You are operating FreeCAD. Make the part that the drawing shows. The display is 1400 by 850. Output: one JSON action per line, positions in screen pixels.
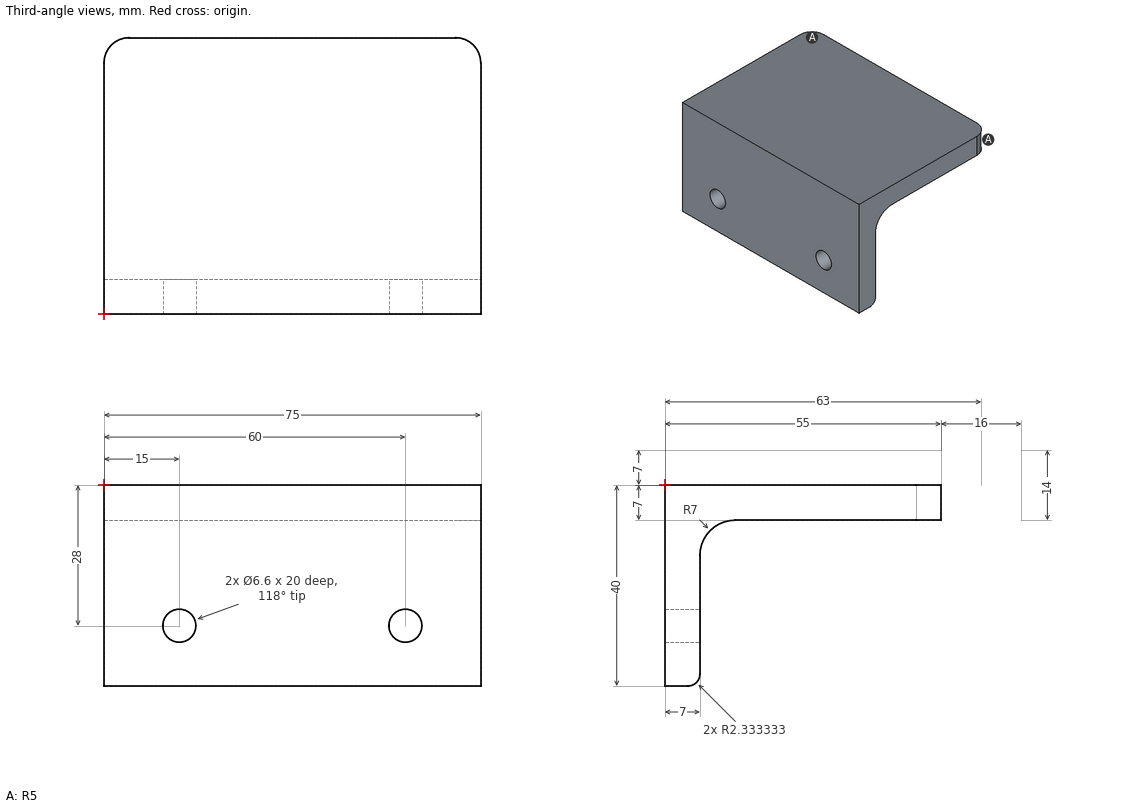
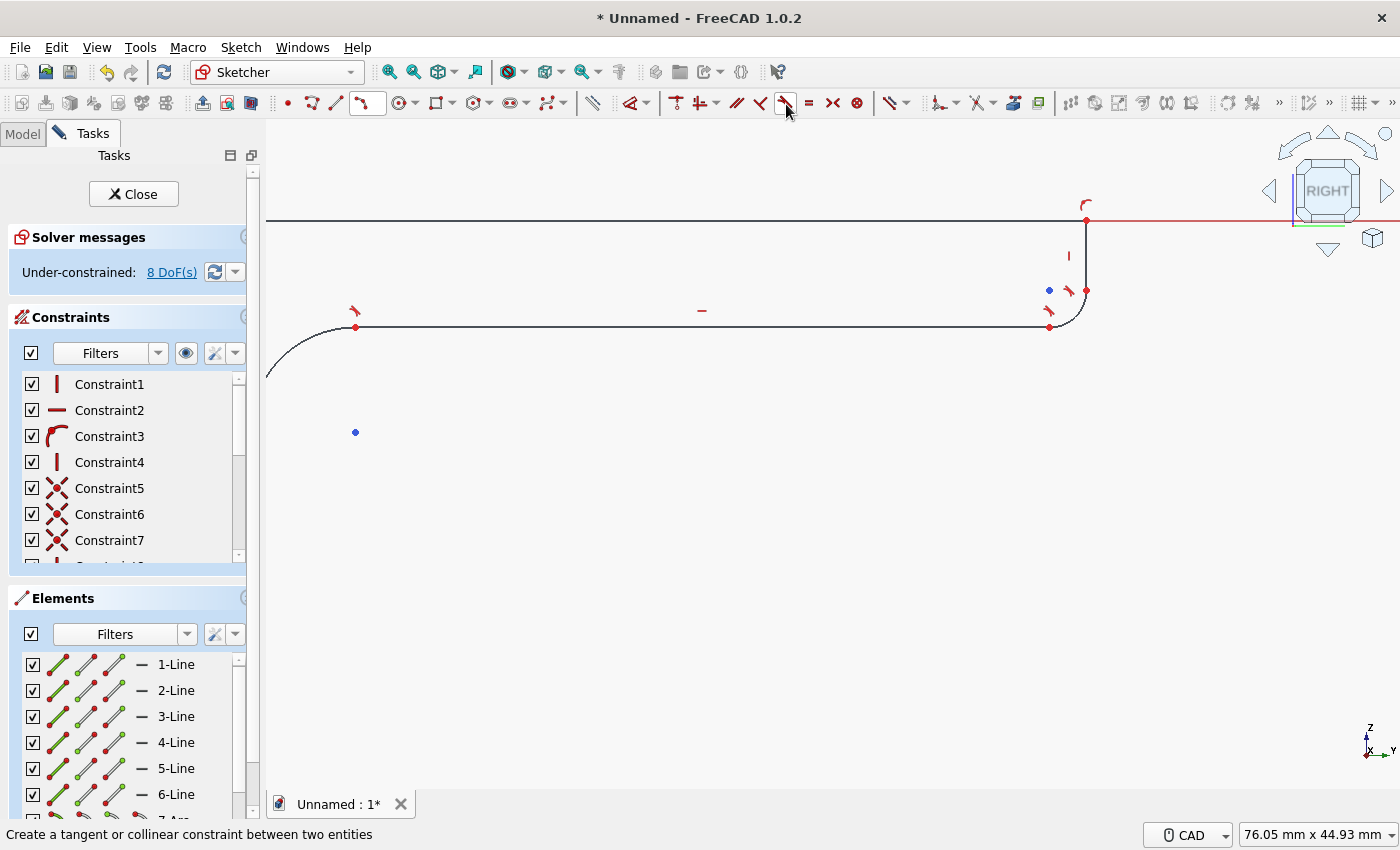
{"action": "scroll", "coordinate": [1066, 322], "scroll_direction": "down", "scroll_amount": 2}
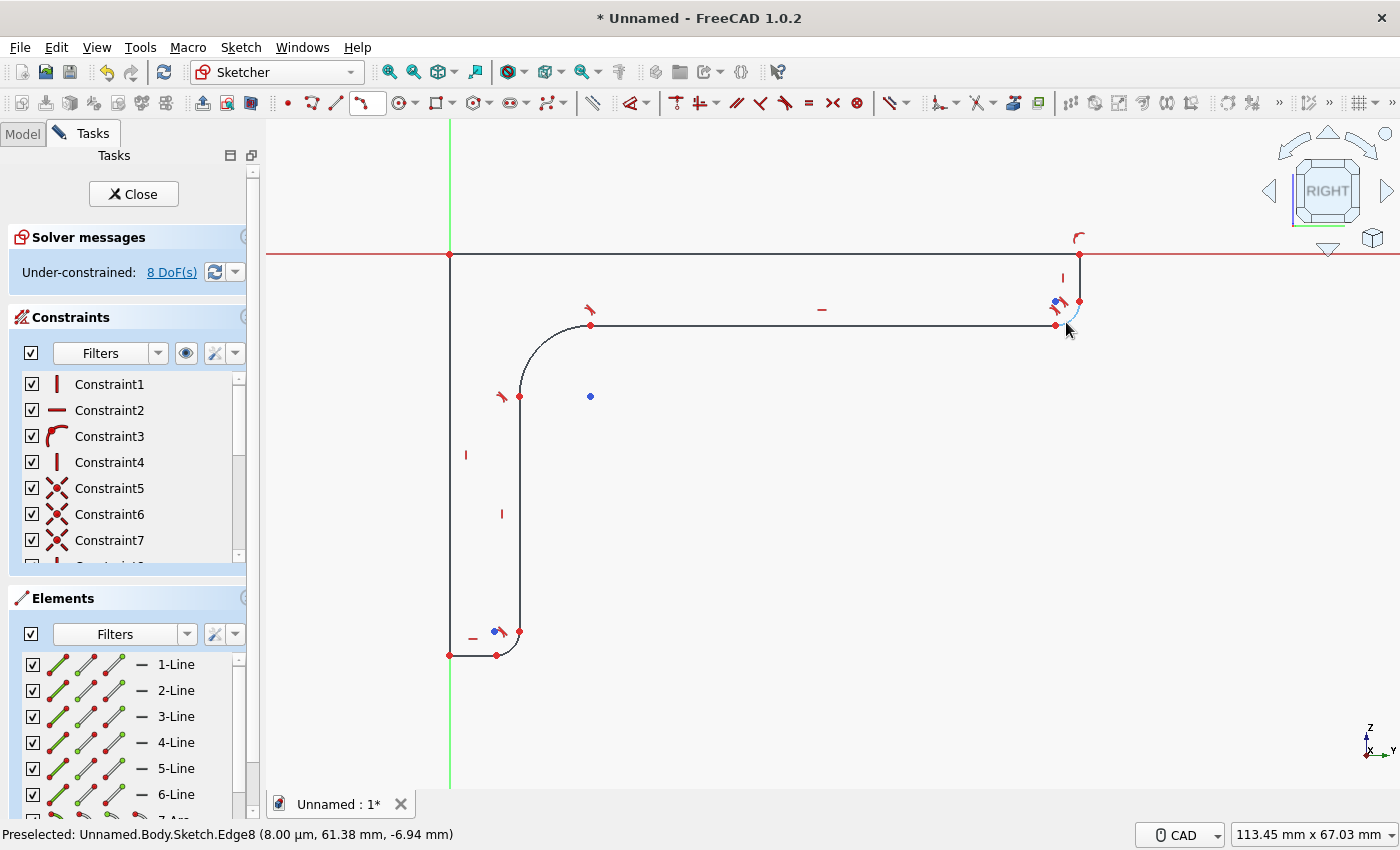
{"action": "left_click", "coordinate": [464, 656]}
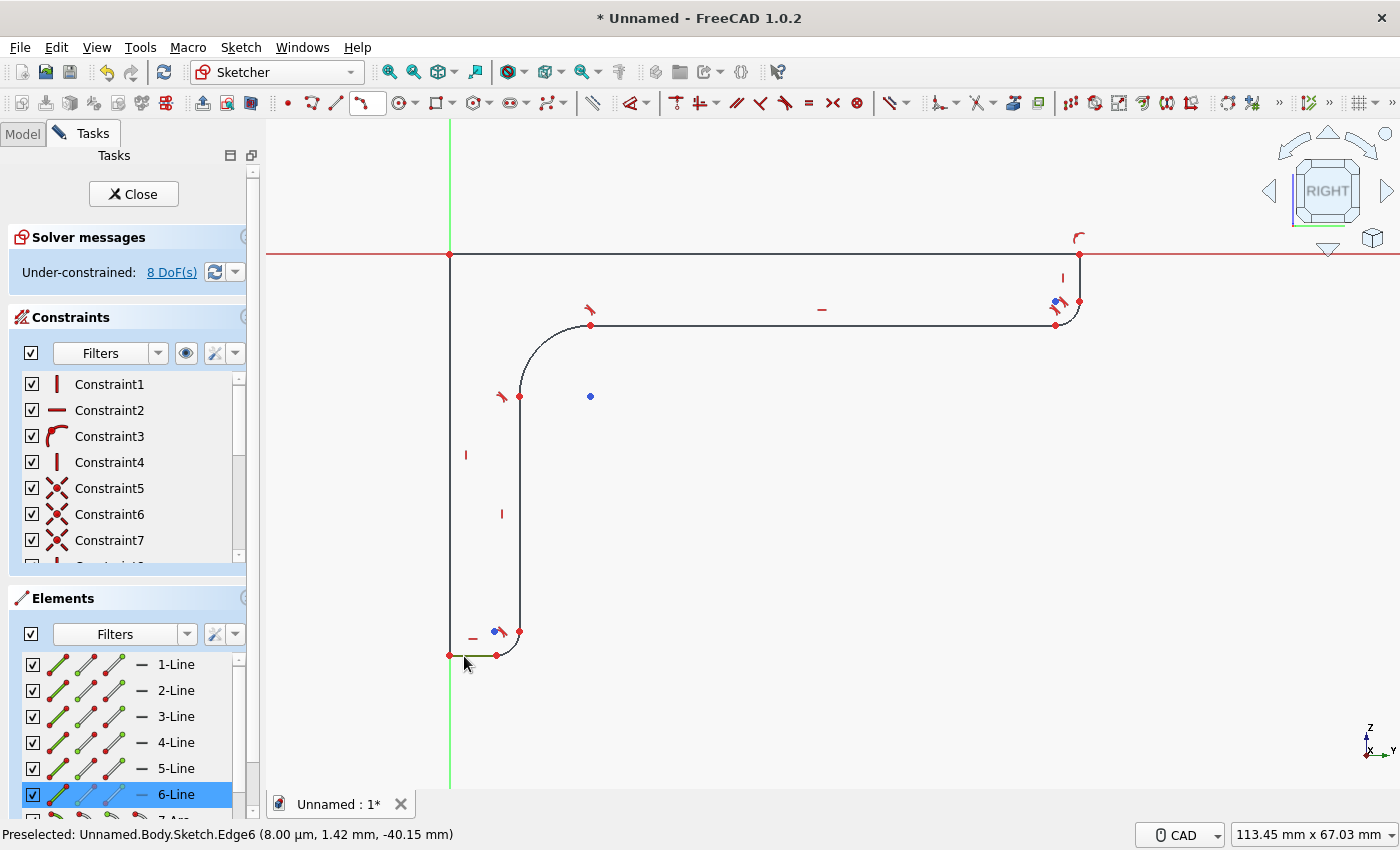
{"action": "scroll", "coordinate": [507, 652], "scroll_direction": "up", "scroll_amount": 2}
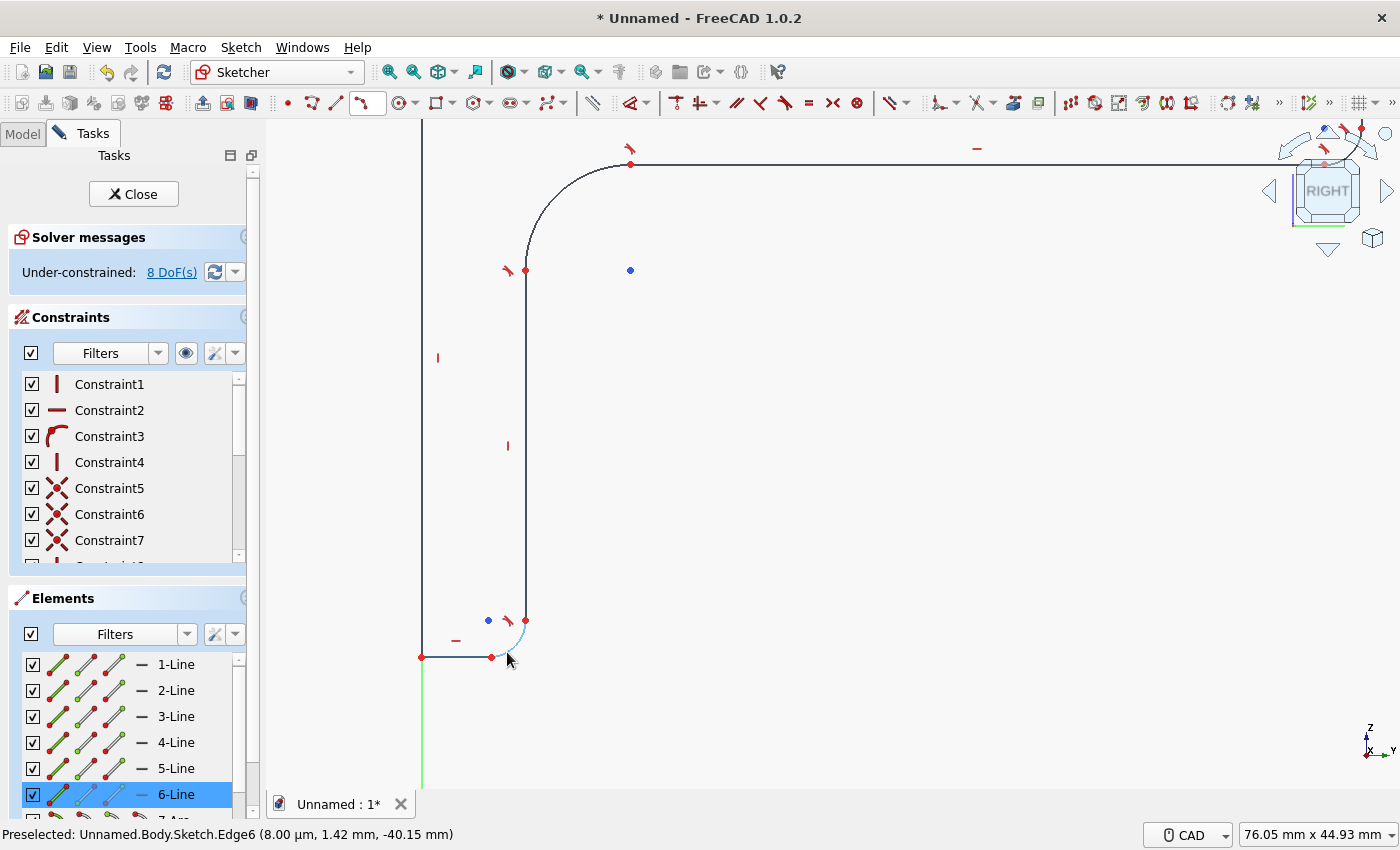
{"action": "left_click", "coordinate": [507, 652]}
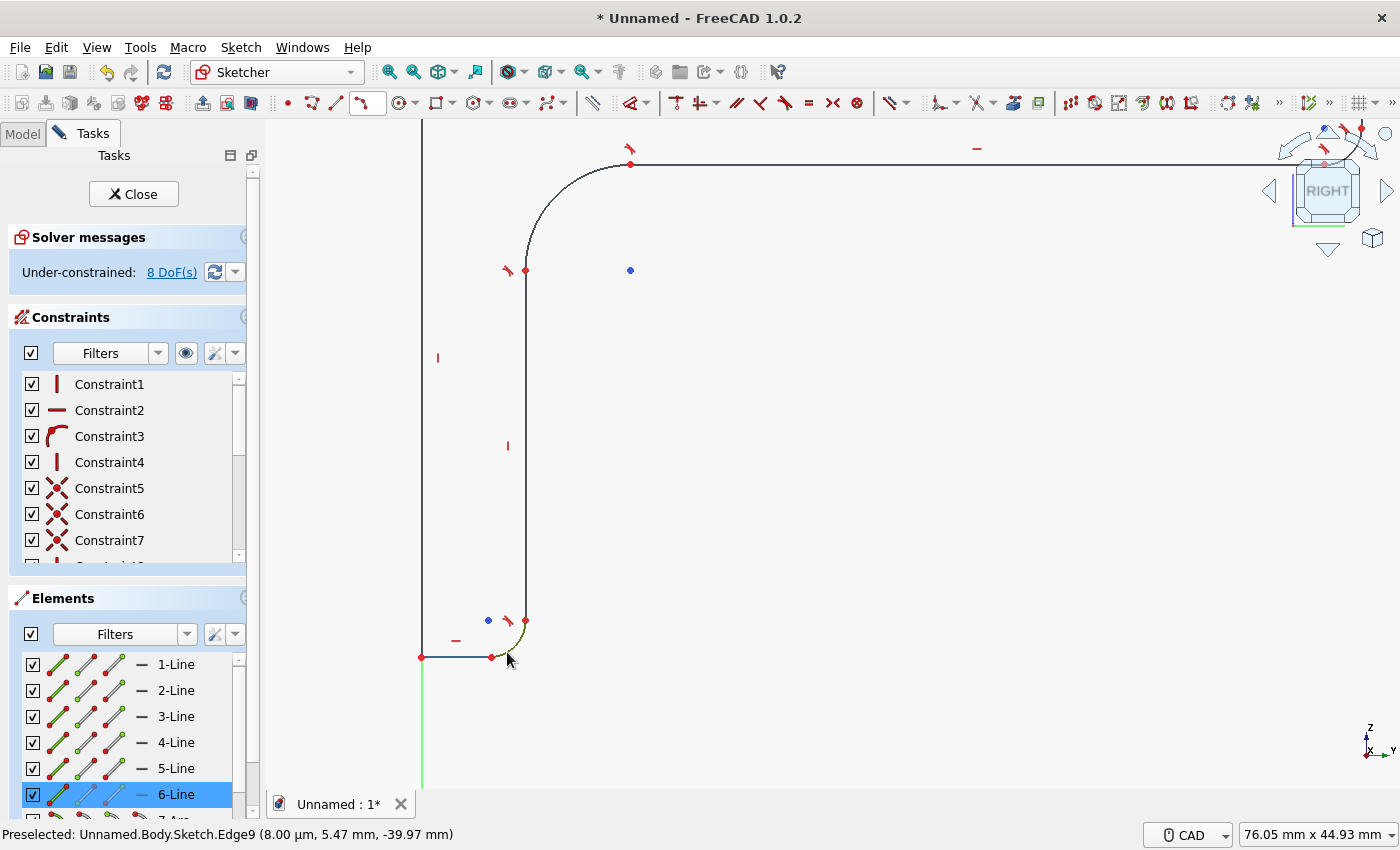
{"action": "key", "text": "t"}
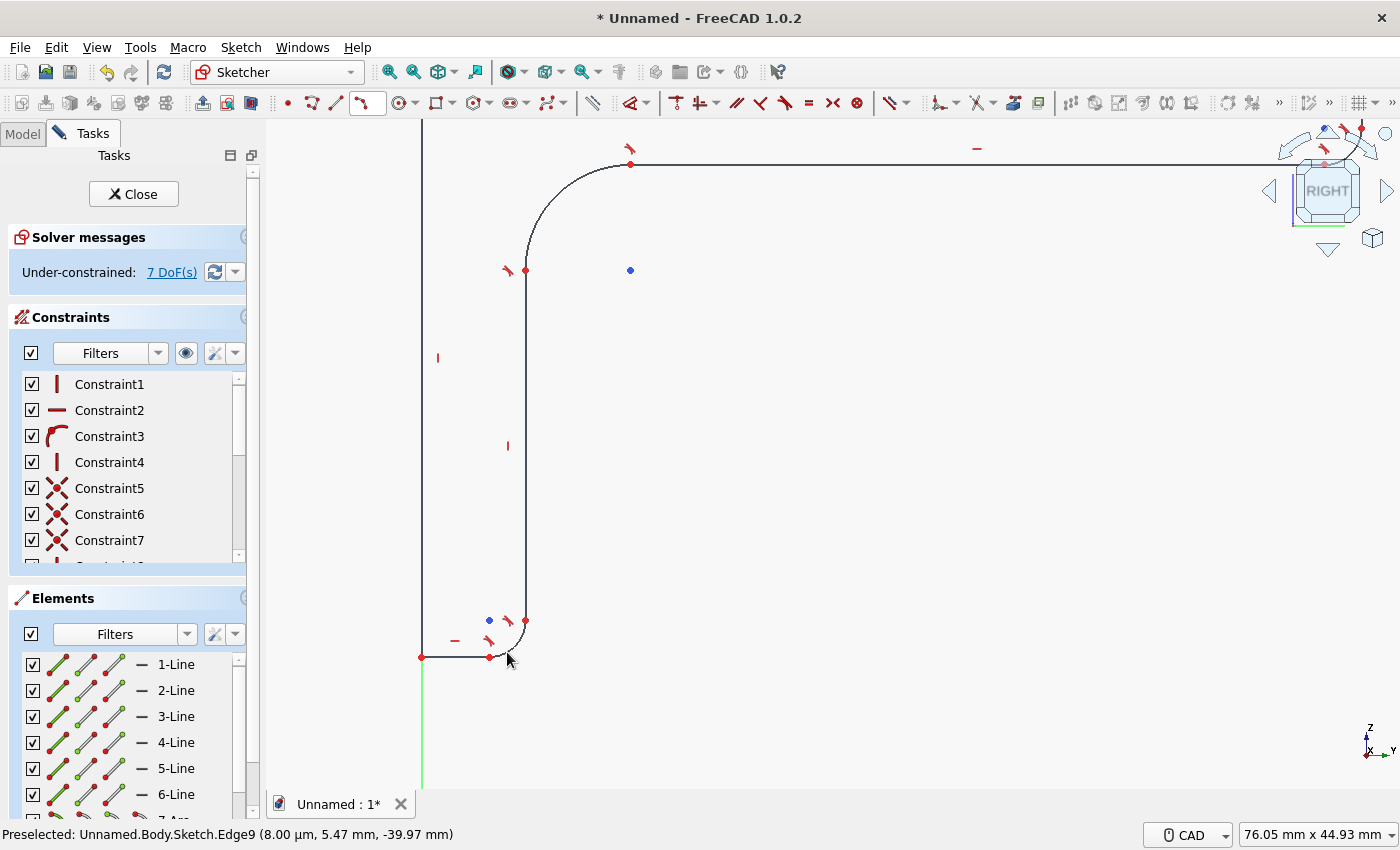
{"action": "scroll", "coordinate": [507, 652], "scroll_direction": "down", "scroll_amount": 2}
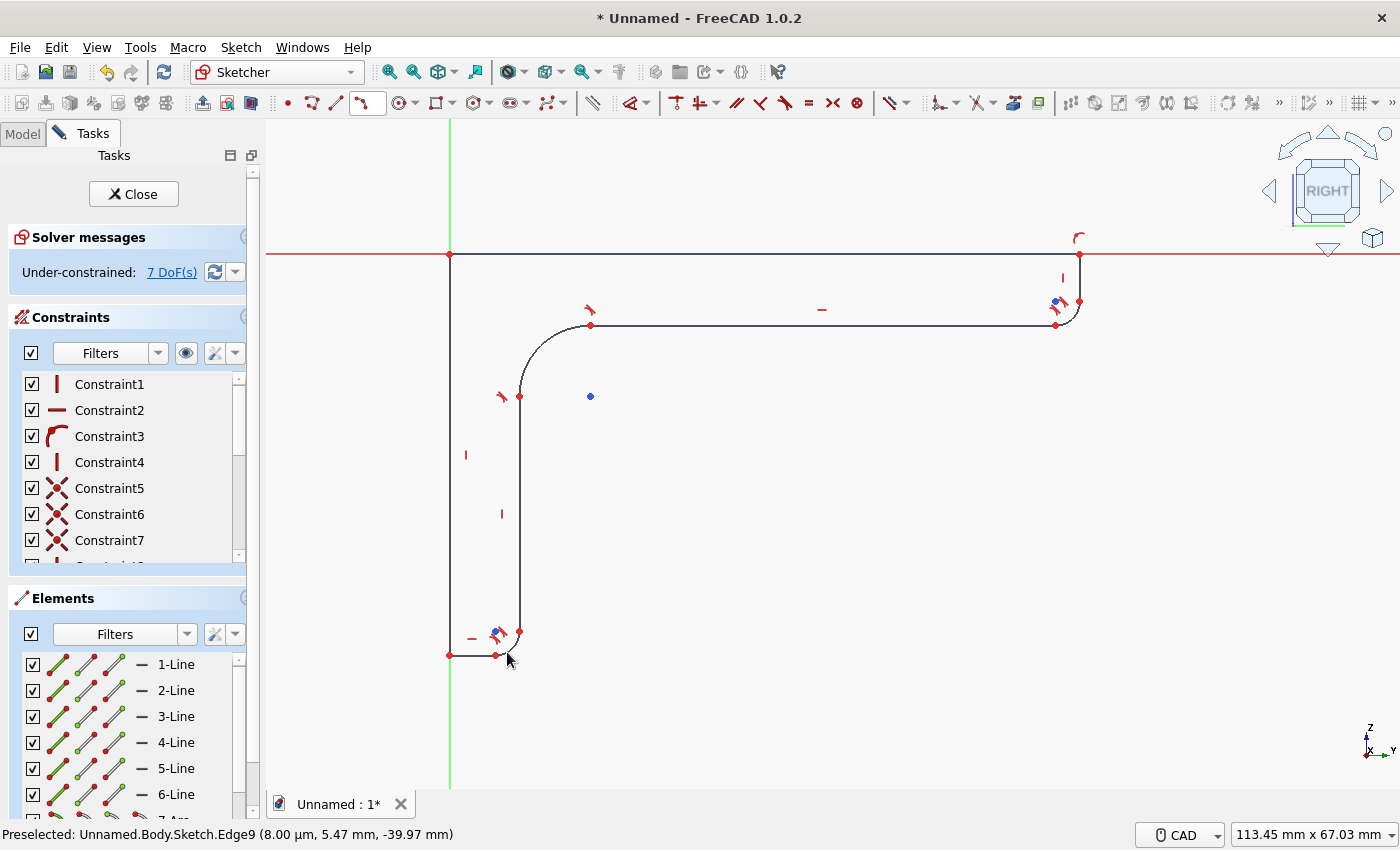
{"action": "left_click", "coordinate": [1066, 323]}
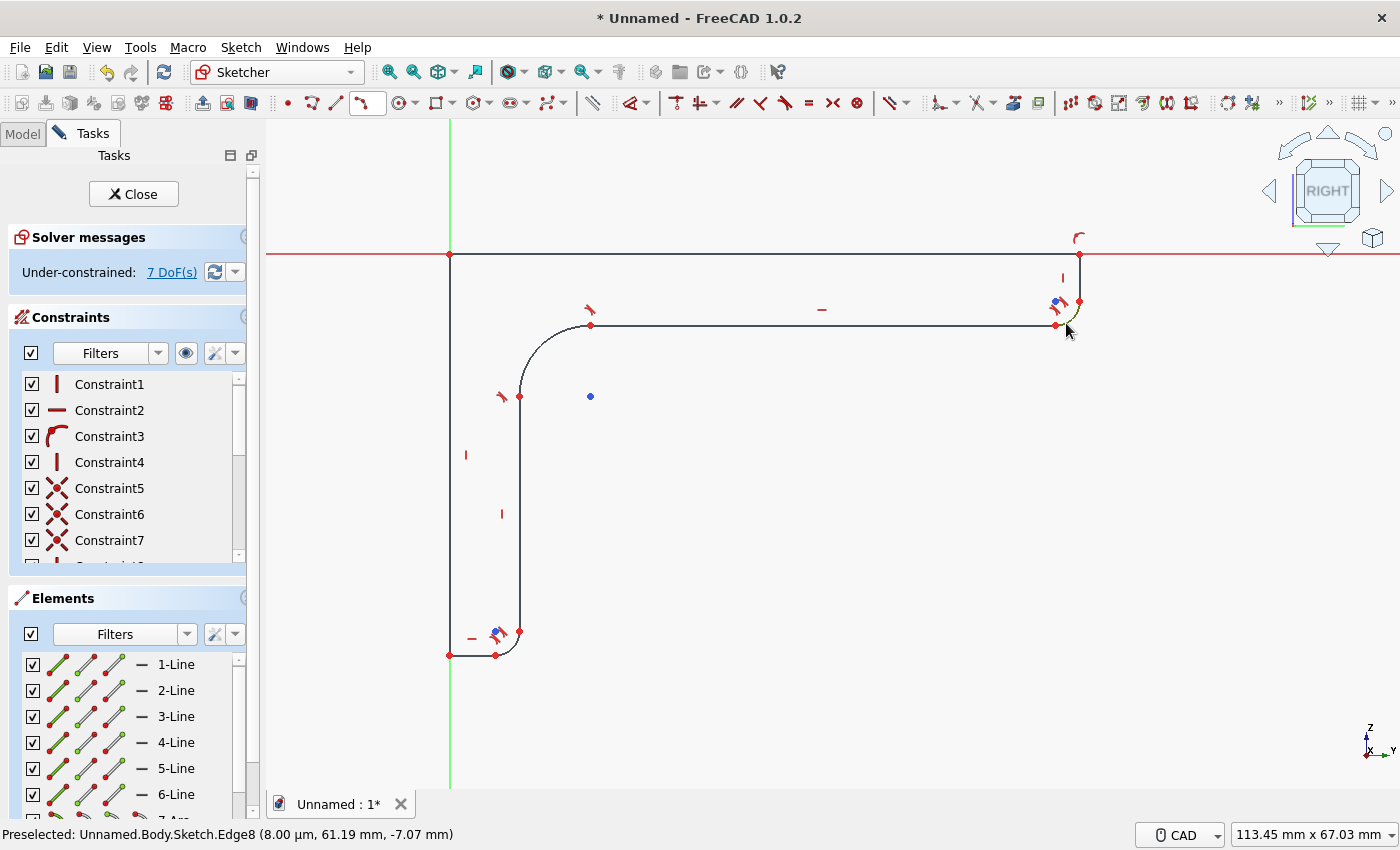
{"action": "left_click", "coordinate": [506, 653]}